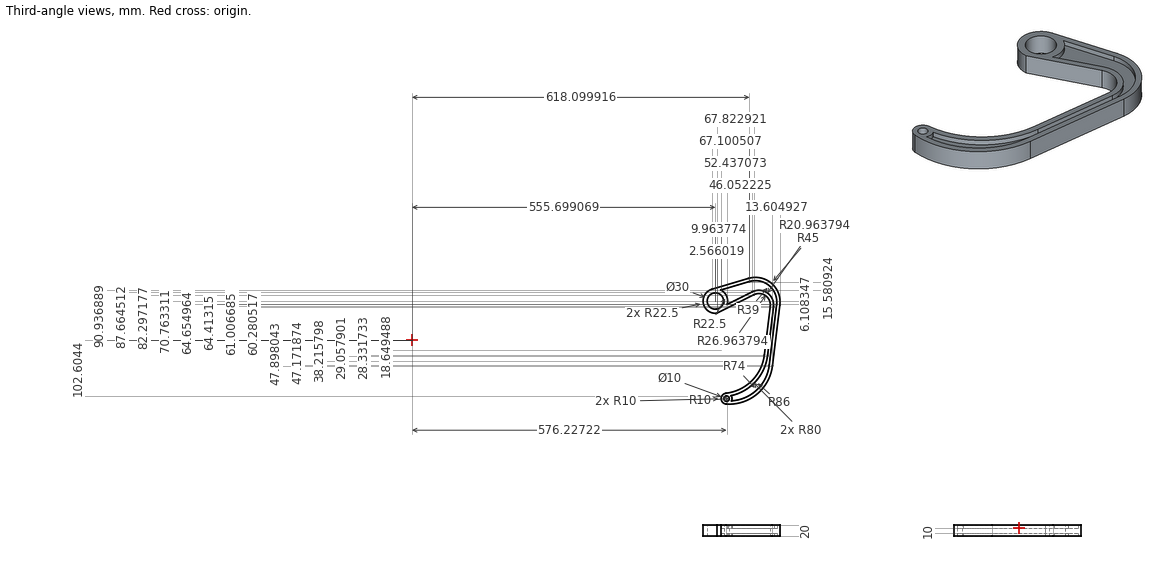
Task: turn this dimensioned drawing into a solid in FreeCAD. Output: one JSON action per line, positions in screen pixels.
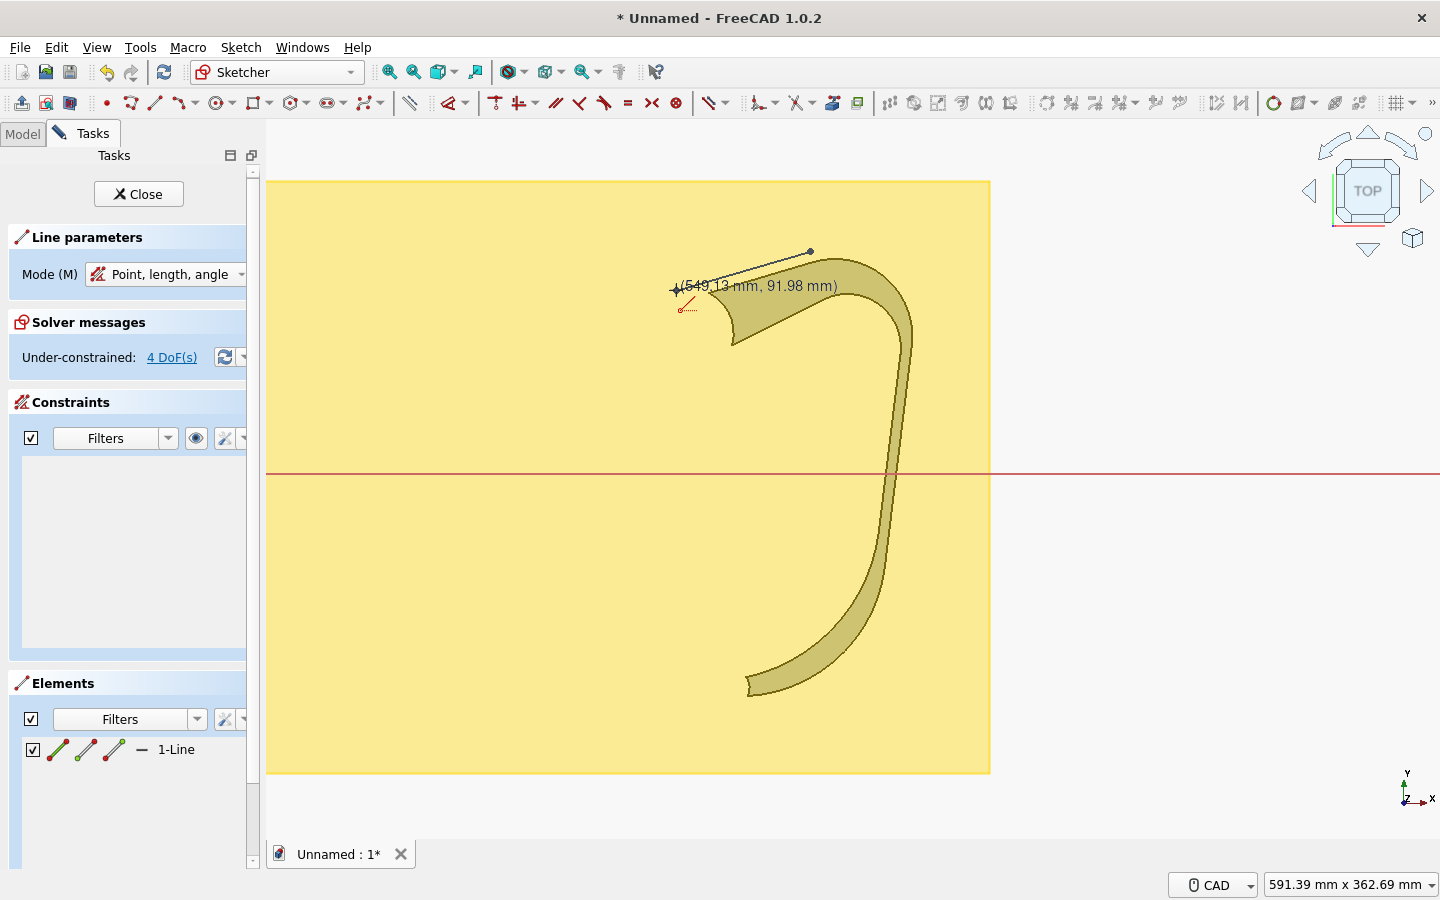
{"action": "left_click", "coordinate": [694, 377]}
{"action": "left_click", "coordinate": [829, 310]}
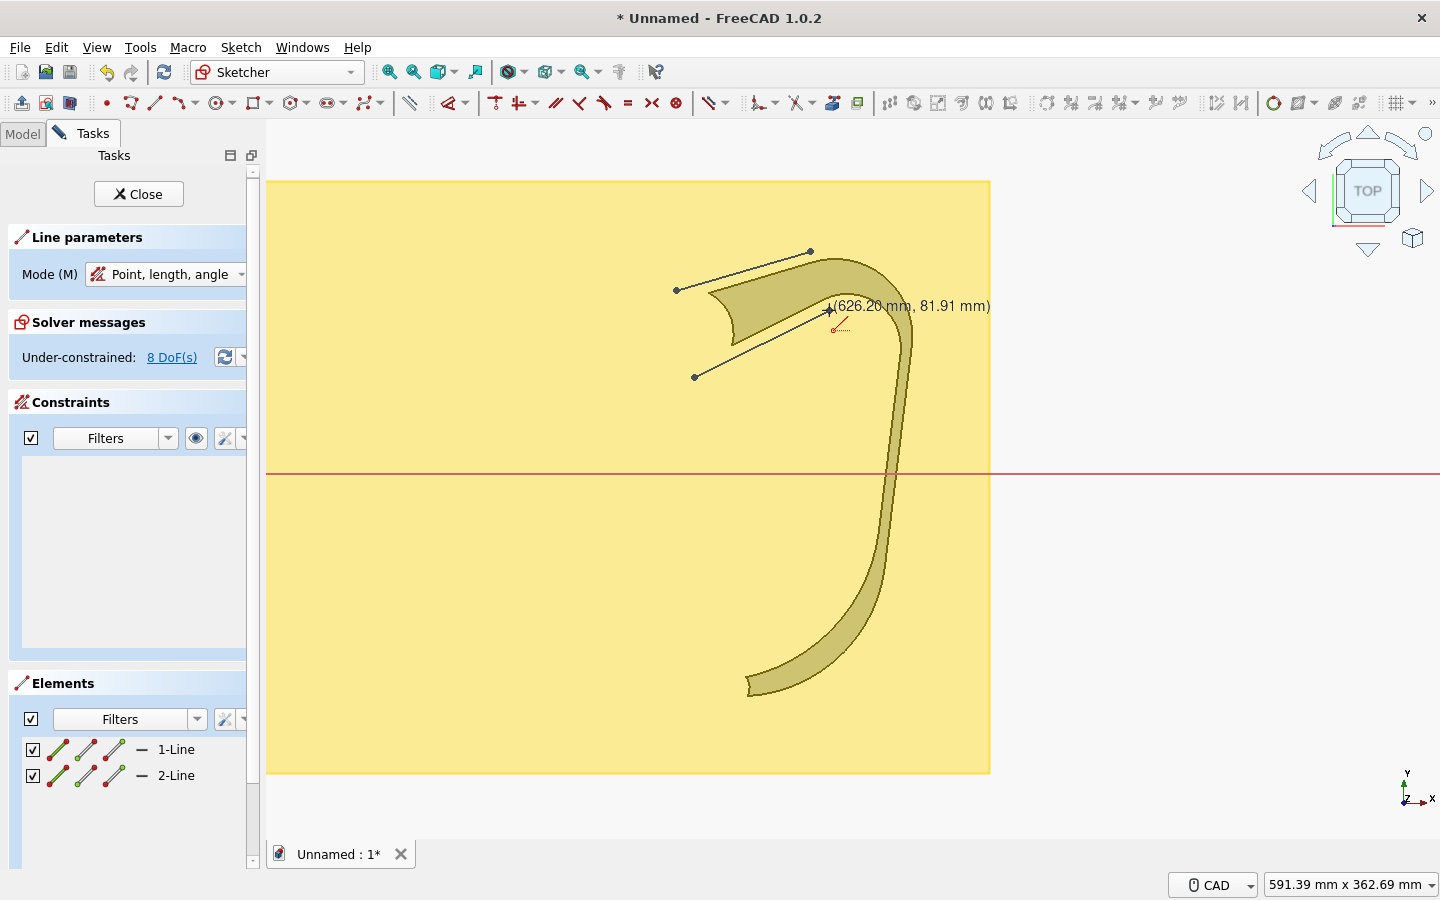
{"action": "left_click", "coordinate": [889, 352]}
{"action": "left_click", "coordinate": [867, 530]}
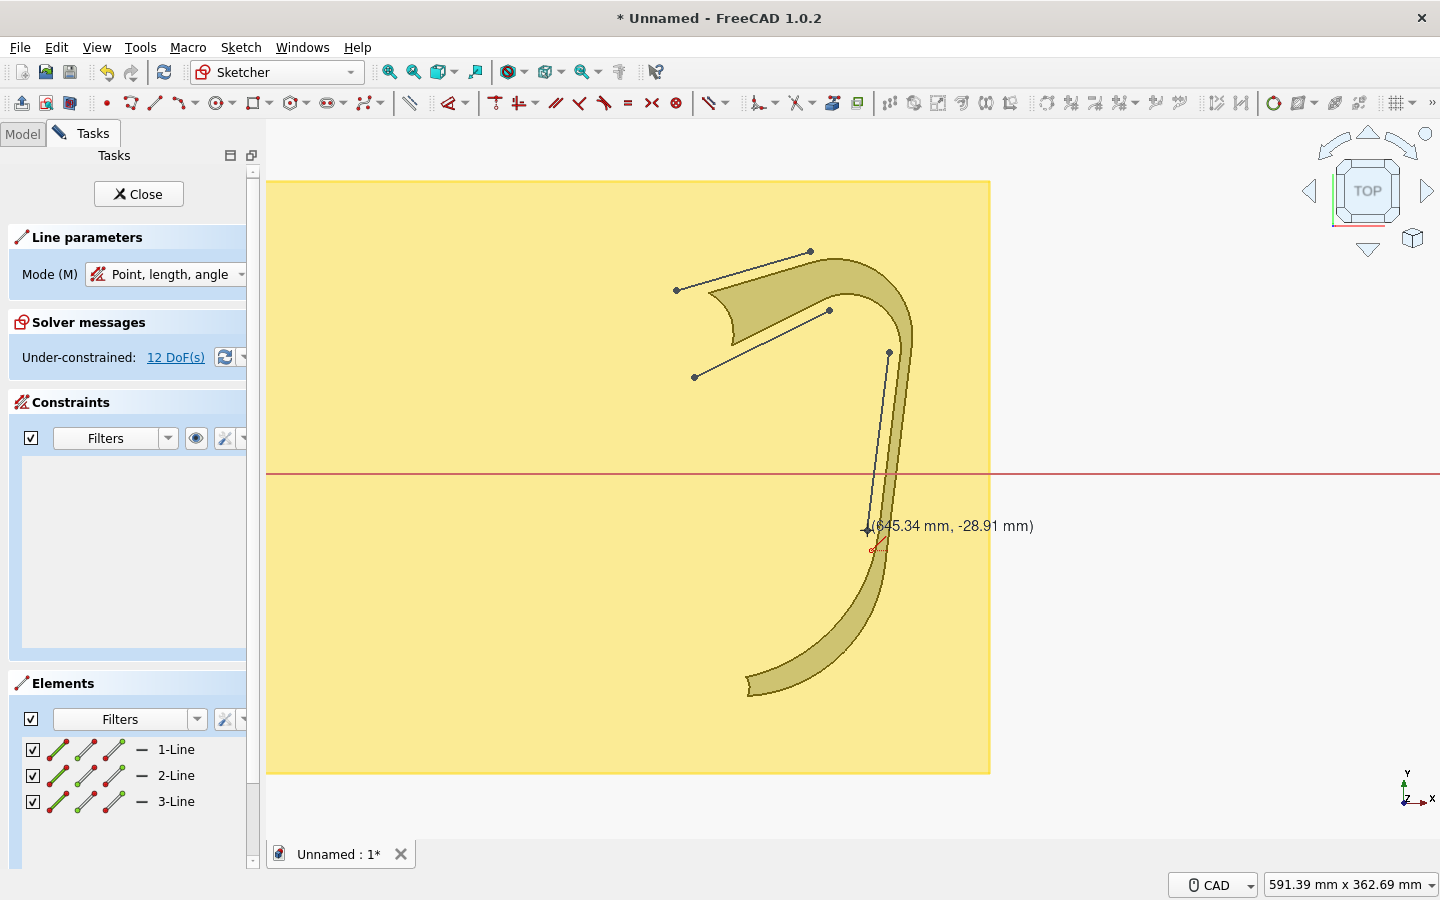
{"action": "left_click", "coordinate": [897, 569]}
{"action": "left_click", "coordinate": [924, 347]}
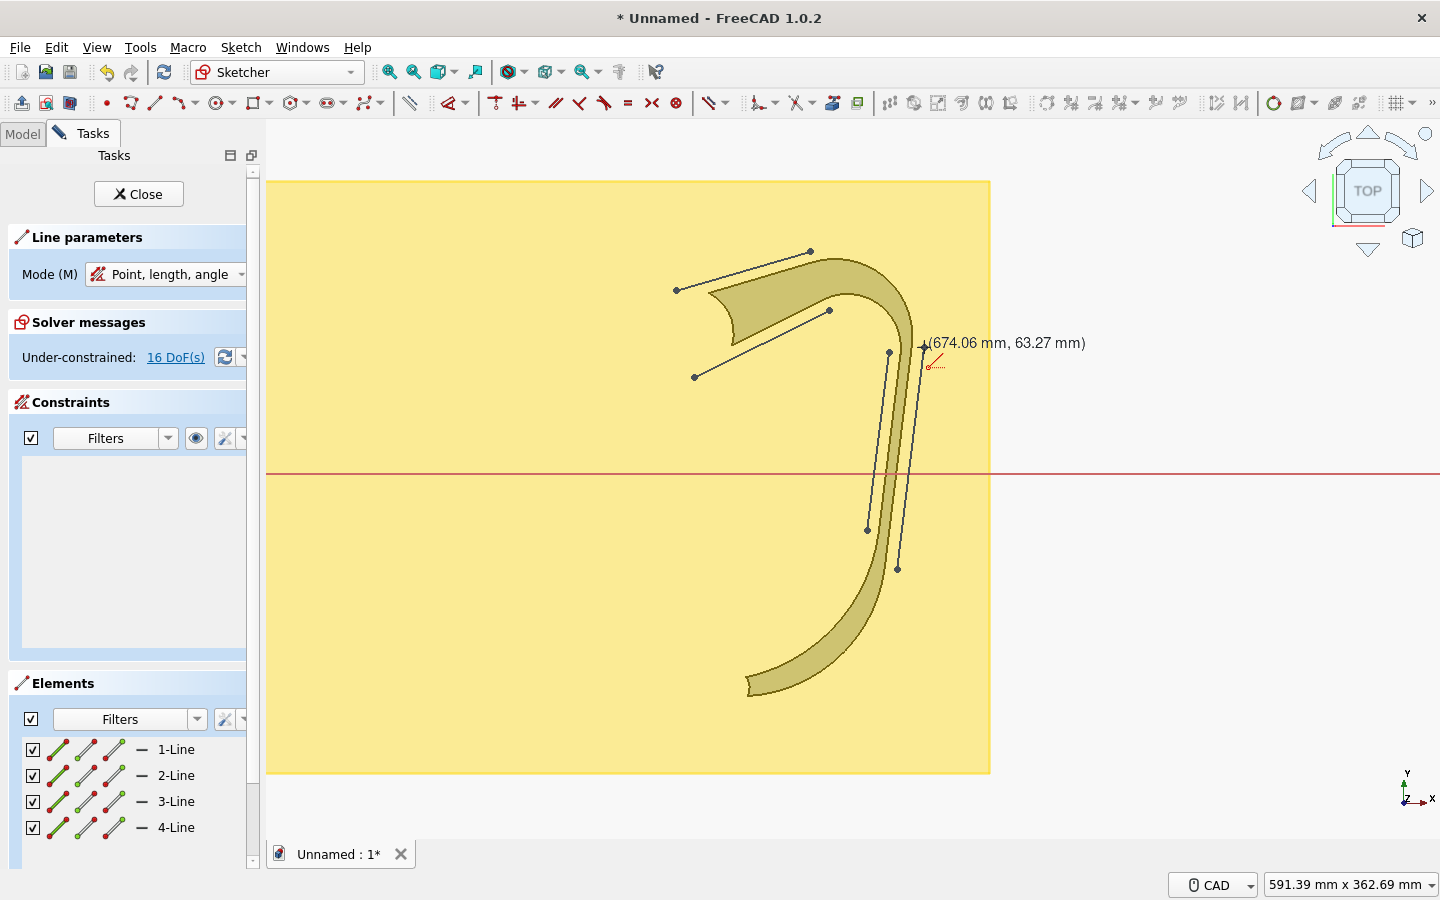
{"action": "left_click", "coordinate": [180, 104]}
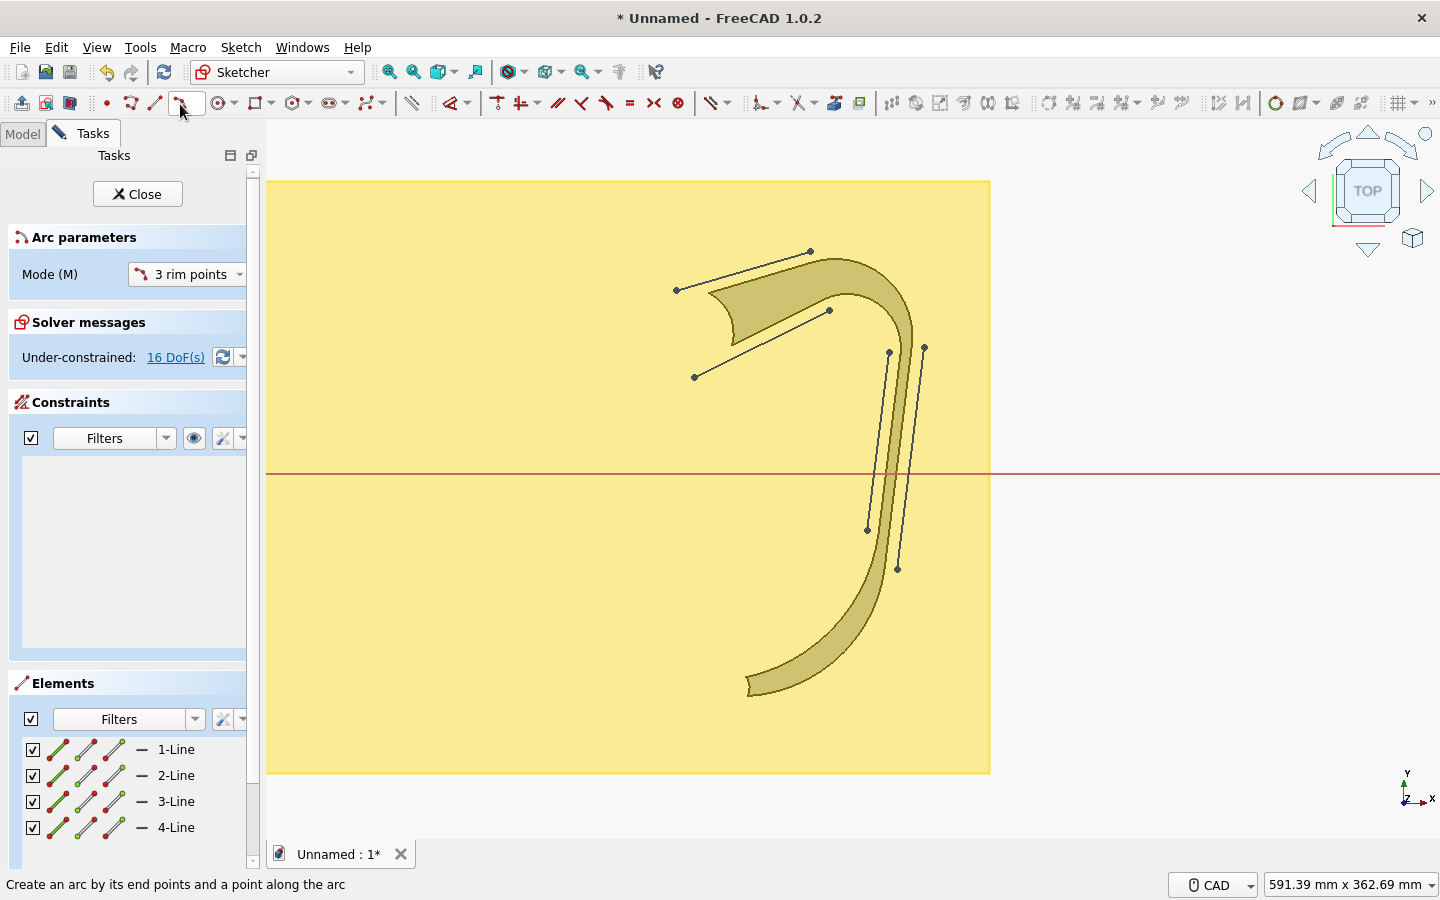
{"action": "left_click", "coordinate": [676, 291]}
{"action": "left_click", "coordinate": [694, 378]}
{"action": "left_click", "coordinate": [645, 342]}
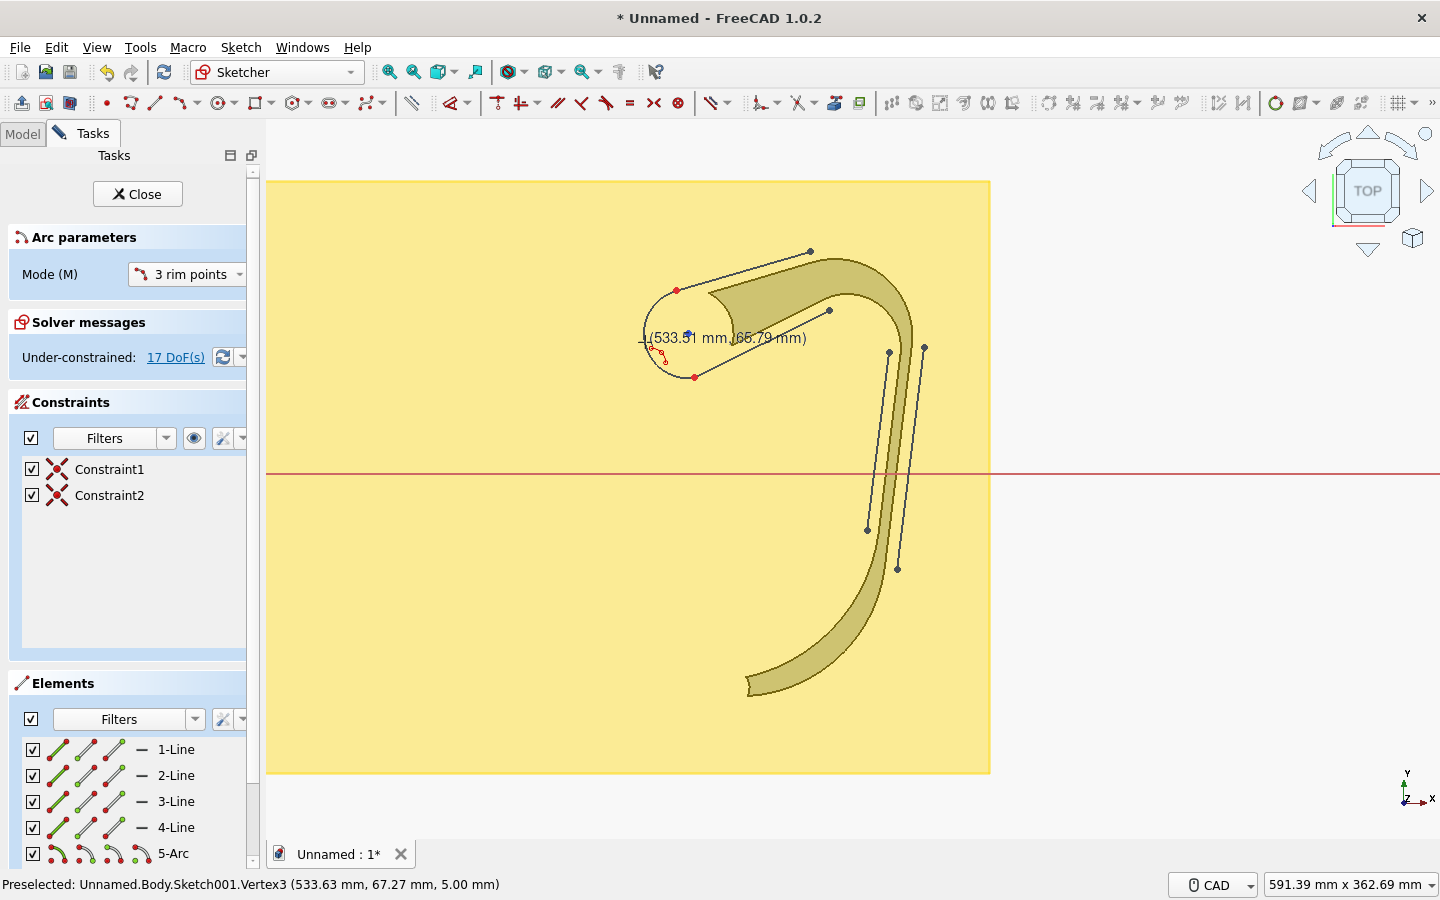
{"action": "left_click", "coordinate": [829, 311]}
{"action": "left_click", "coordinate": [889, 353]}
{"action": "left_click", "coordinate": [871, 313]}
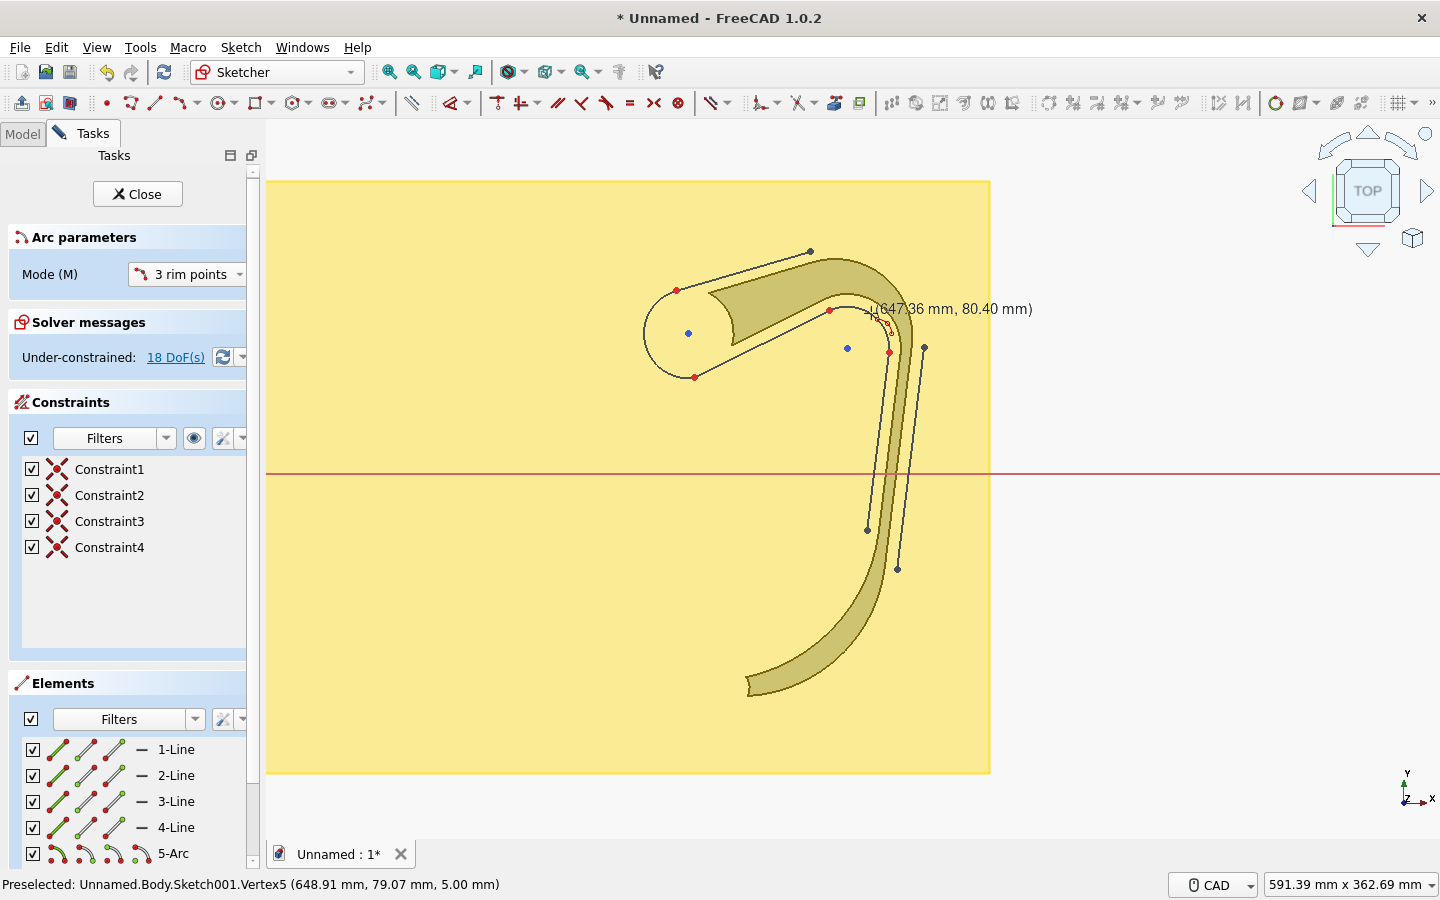
{"action": "left_click", "coordinate": [867, 531]}
{"action": "left_click", "coordinate": [728, 668]}
{"action": "left_click", "coordinate": [821, 623]}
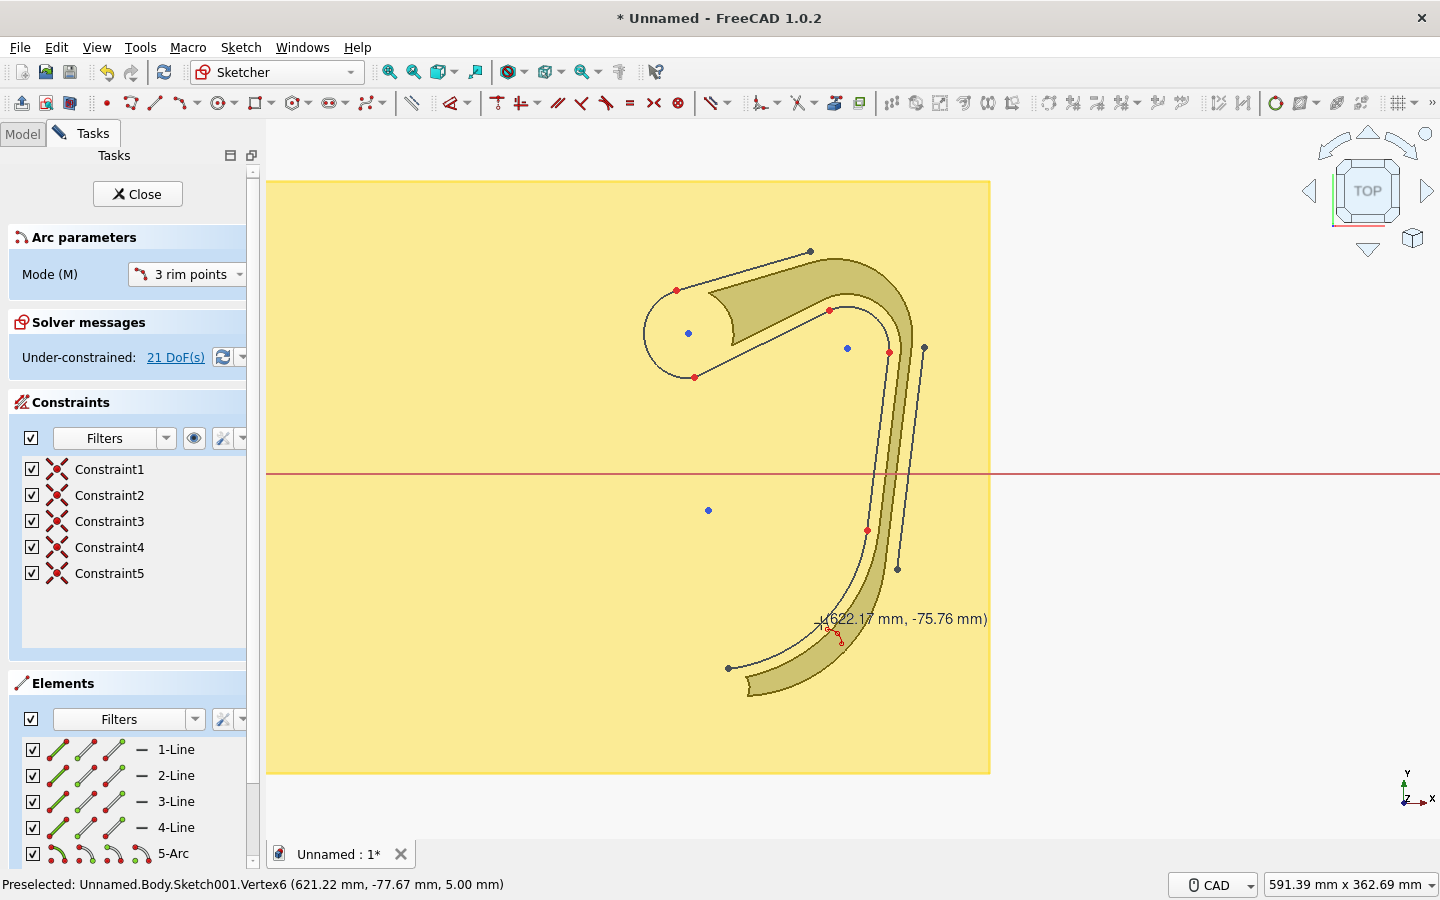
{"action": "left_click", "coordinate": [728, 669]}
{"action": "left_click", "coordinate": [728, 708]}
{"action": "left_click", "coordinate": [710, 689]}